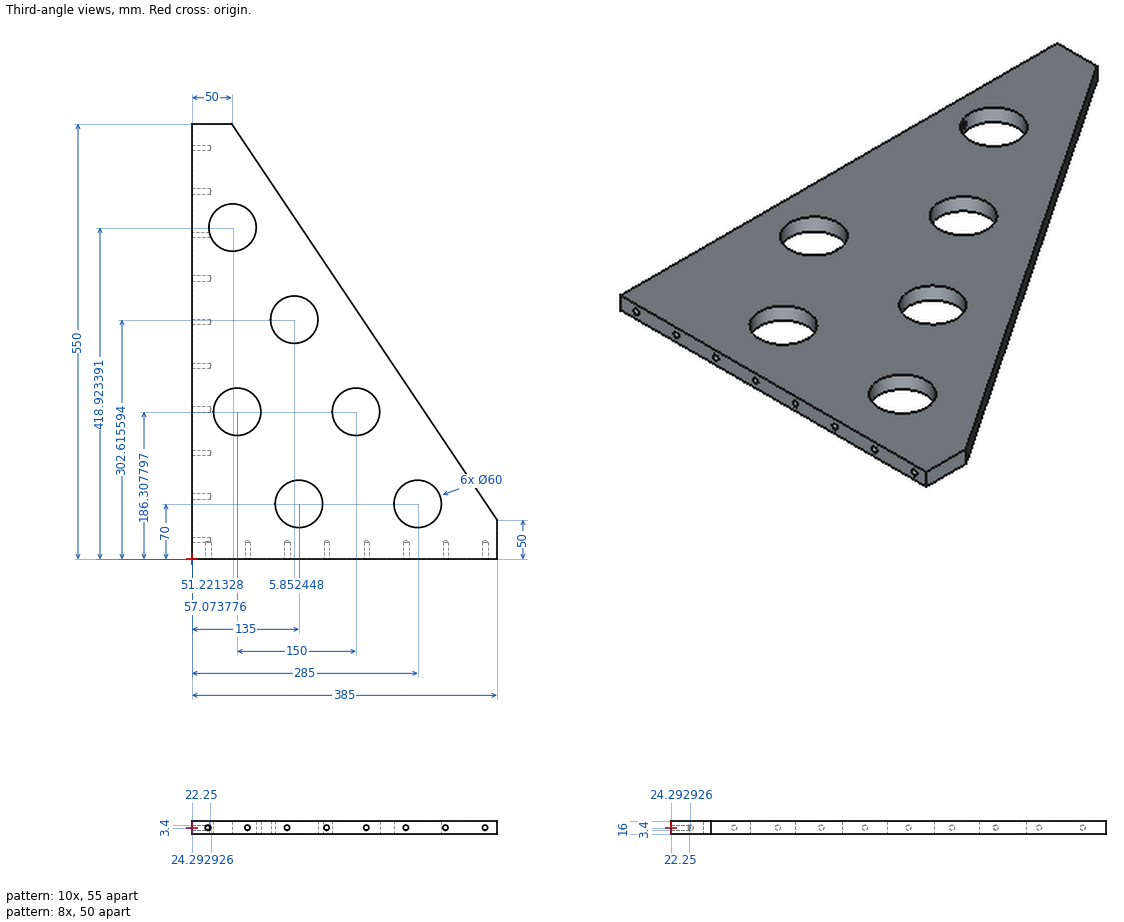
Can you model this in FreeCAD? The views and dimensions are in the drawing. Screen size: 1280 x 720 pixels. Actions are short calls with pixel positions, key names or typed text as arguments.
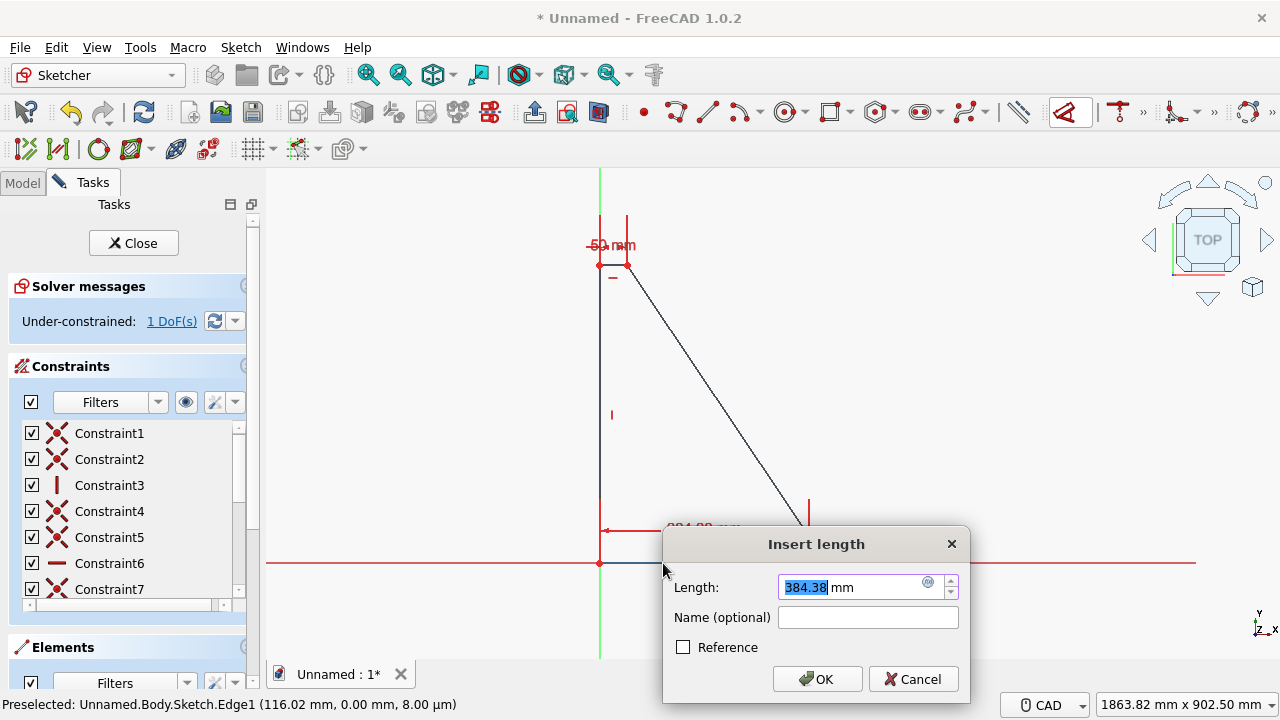
text(385)
key(Return)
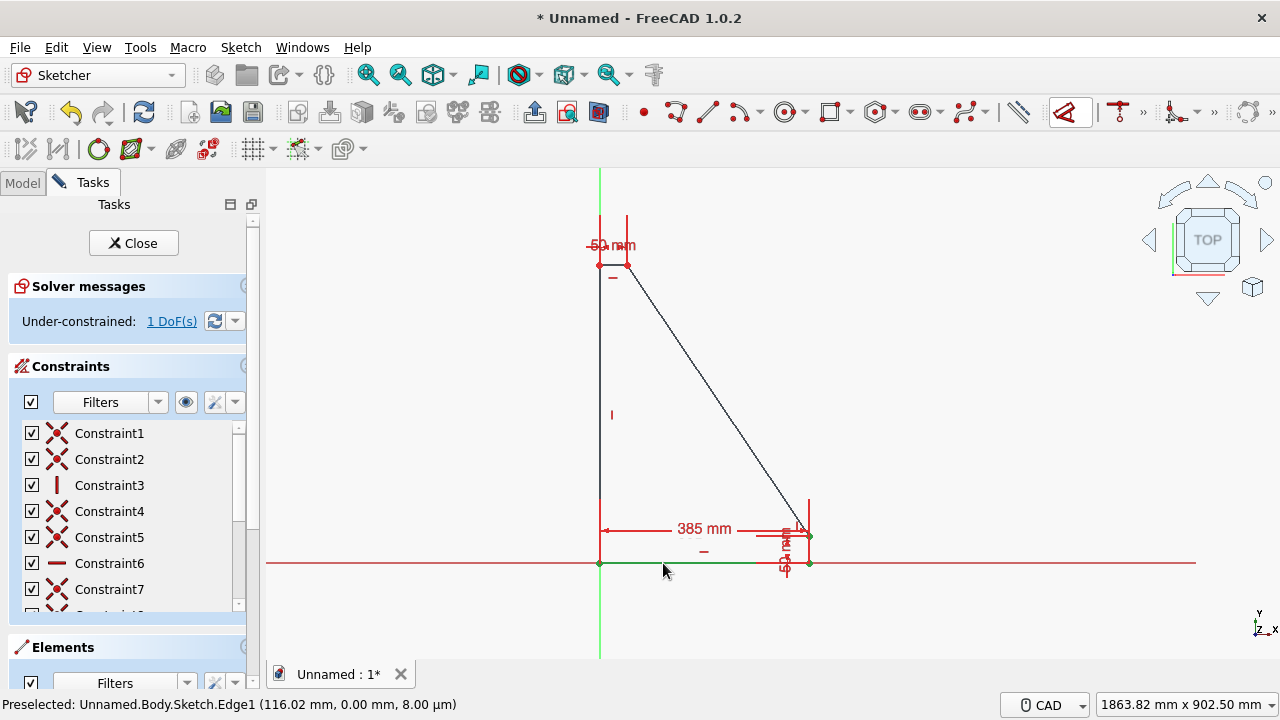
click(600, 355)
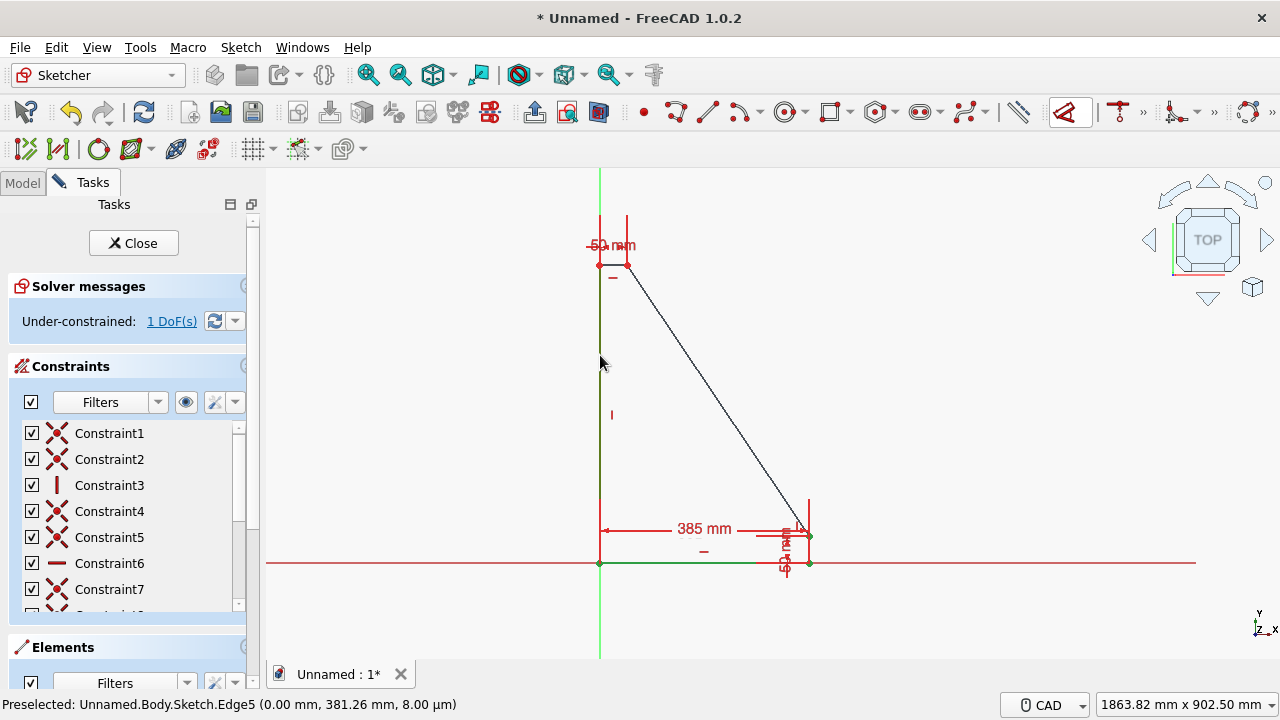
click(1086, 112)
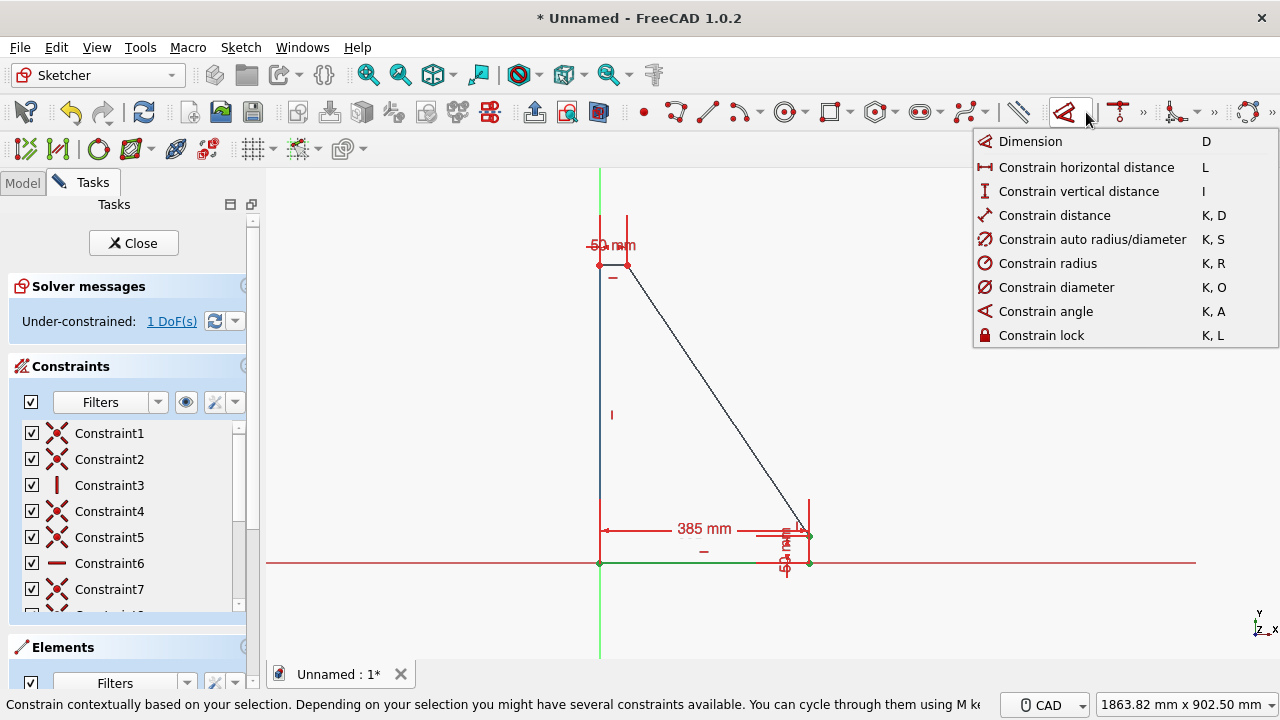
click(1126, 191)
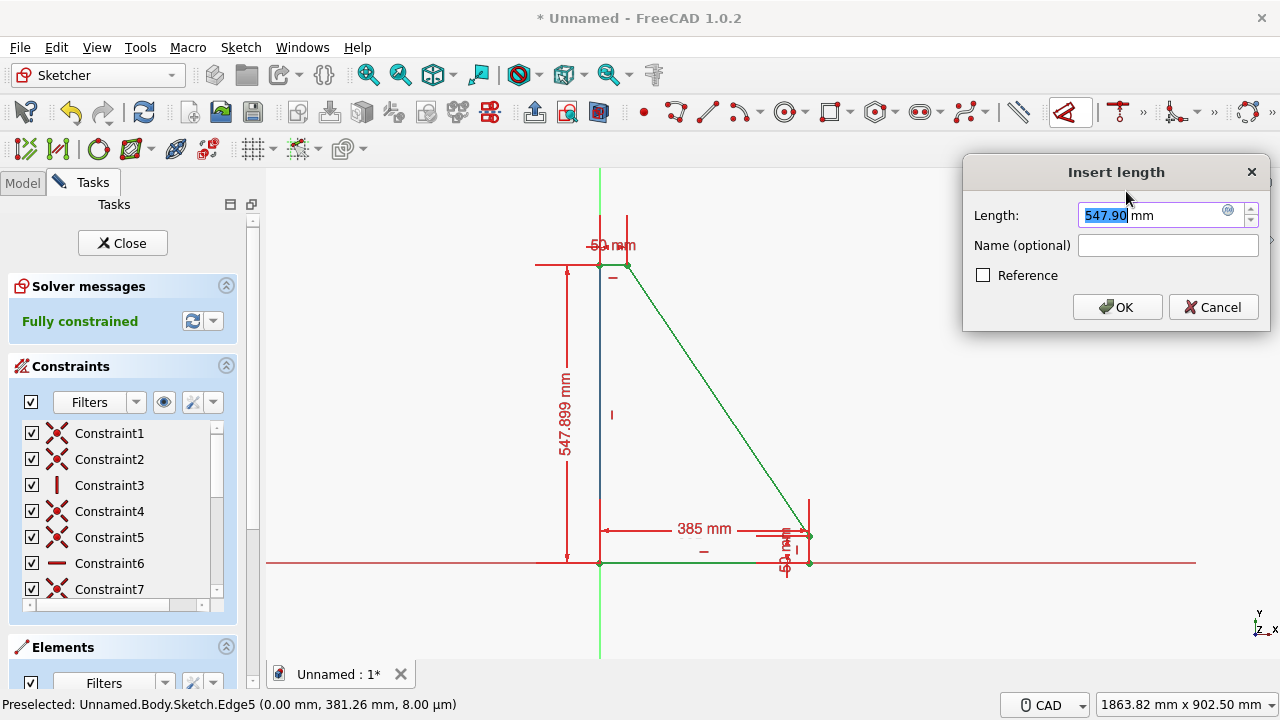
text(550)
key(Return)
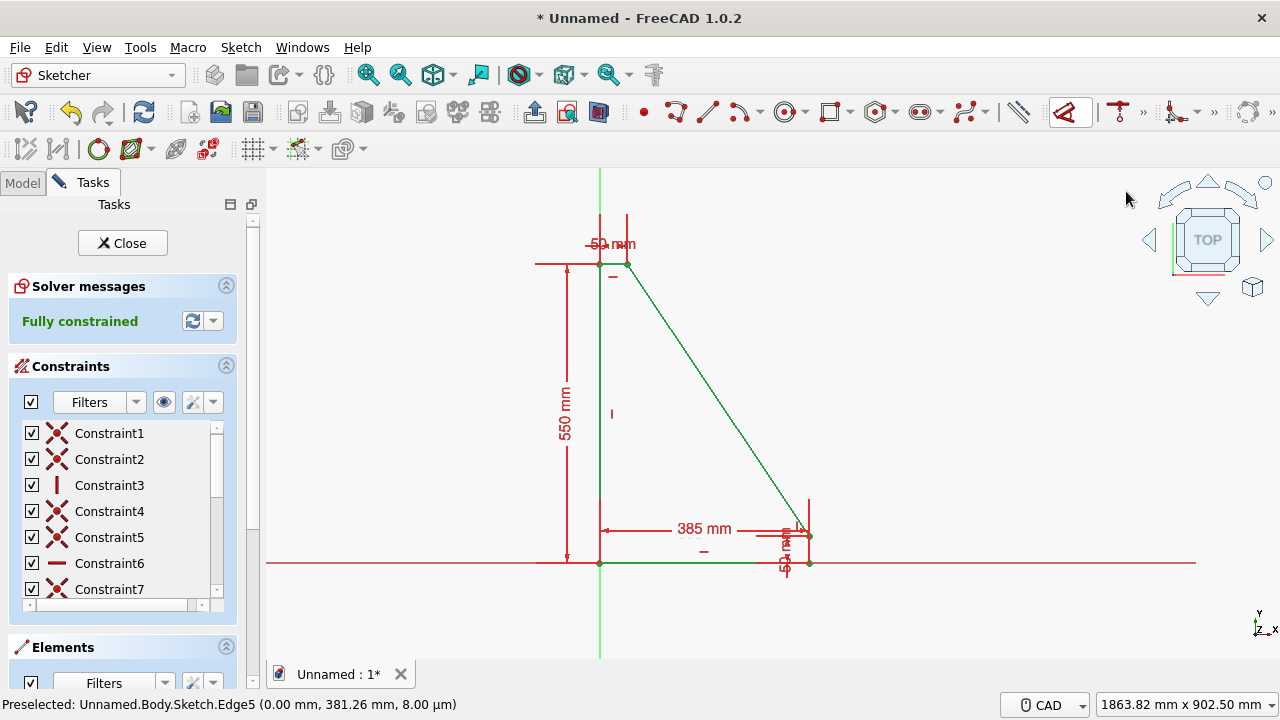
click(123, 243)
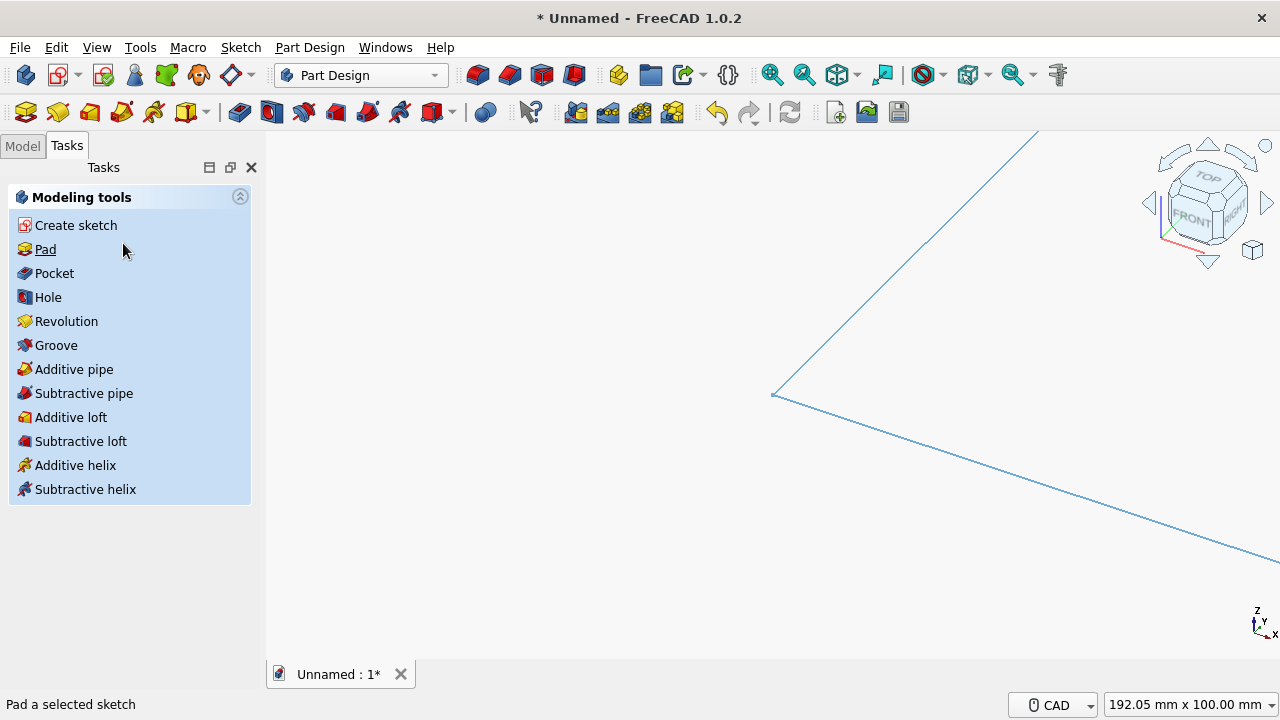
click(26, 112)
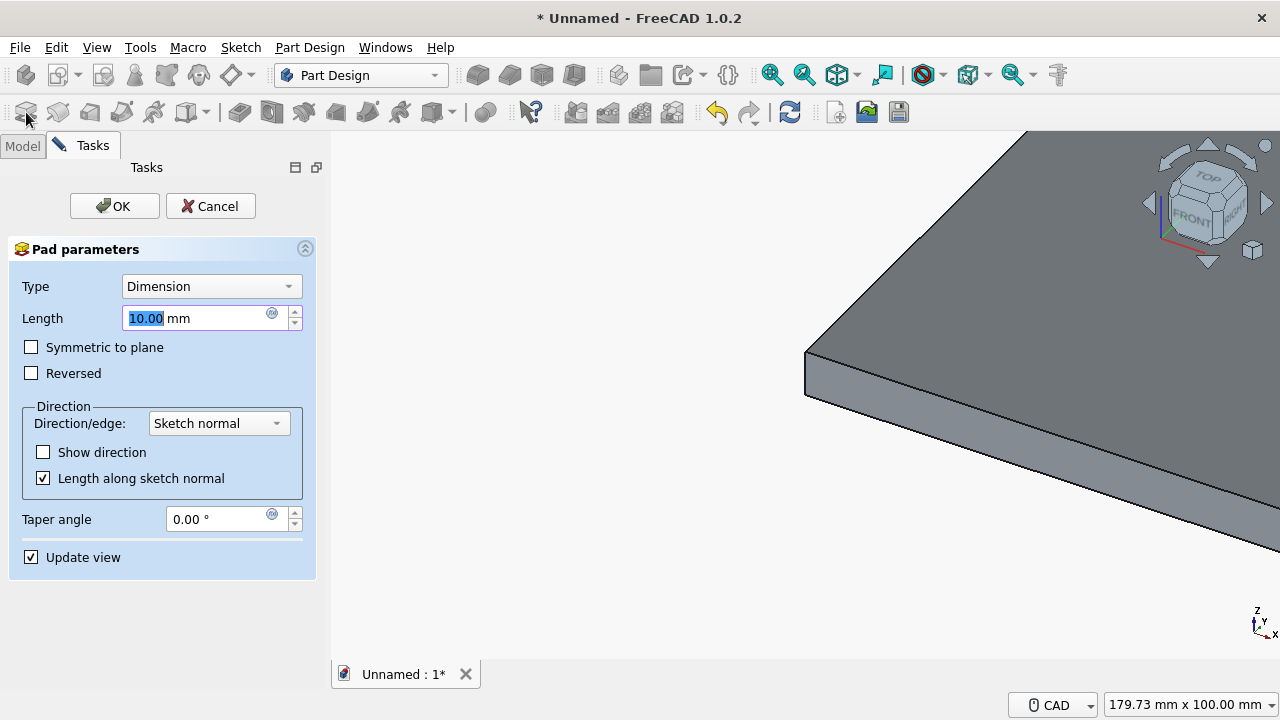
text(16)
key(Tab)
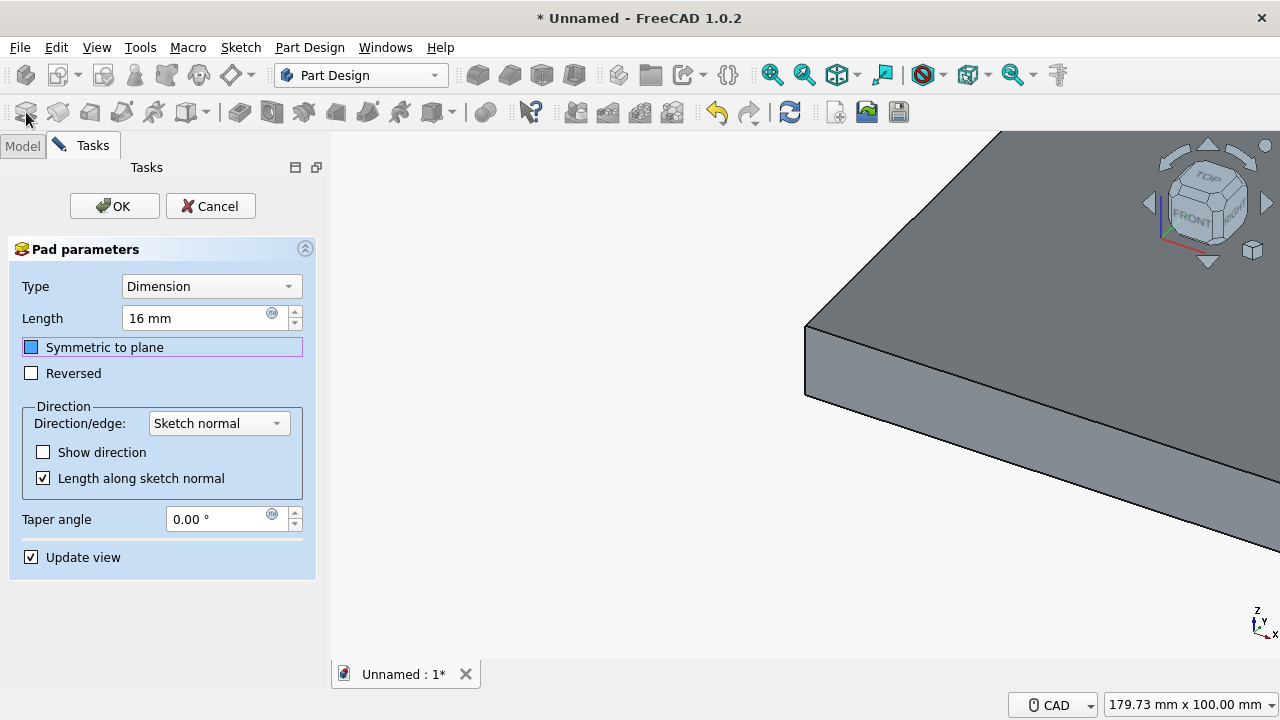
click(30, 347)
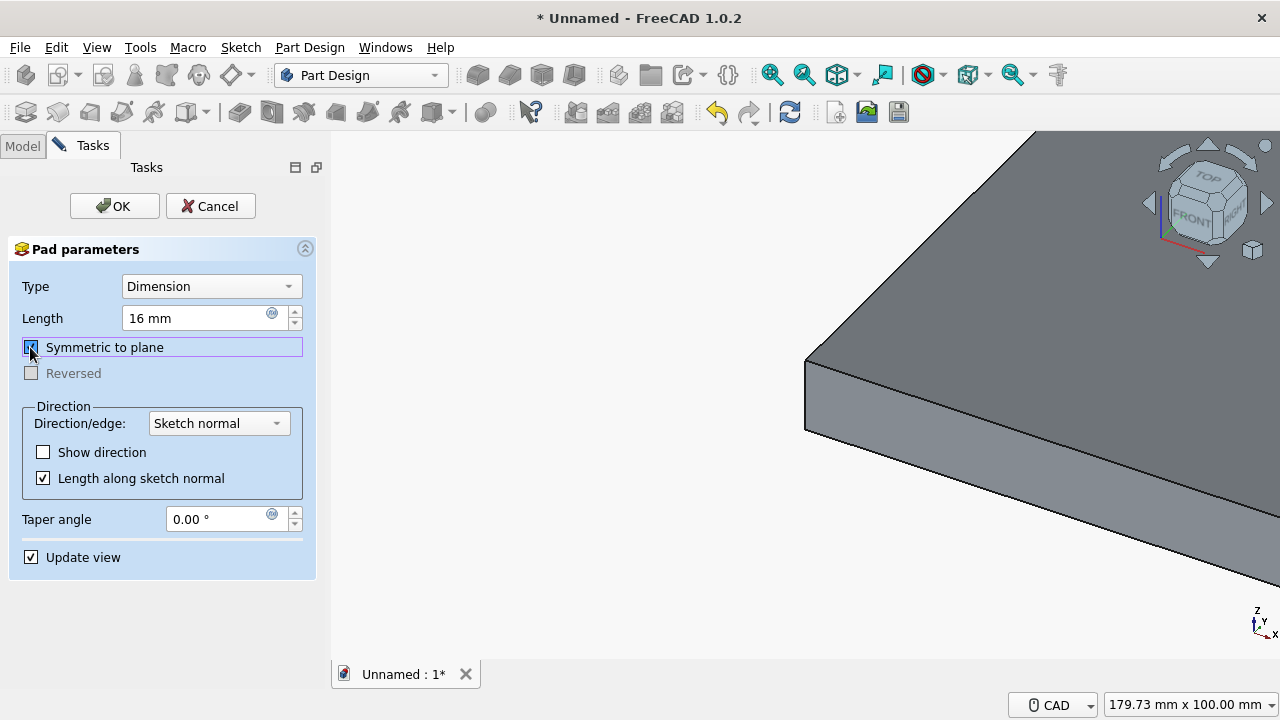
click(115, 206)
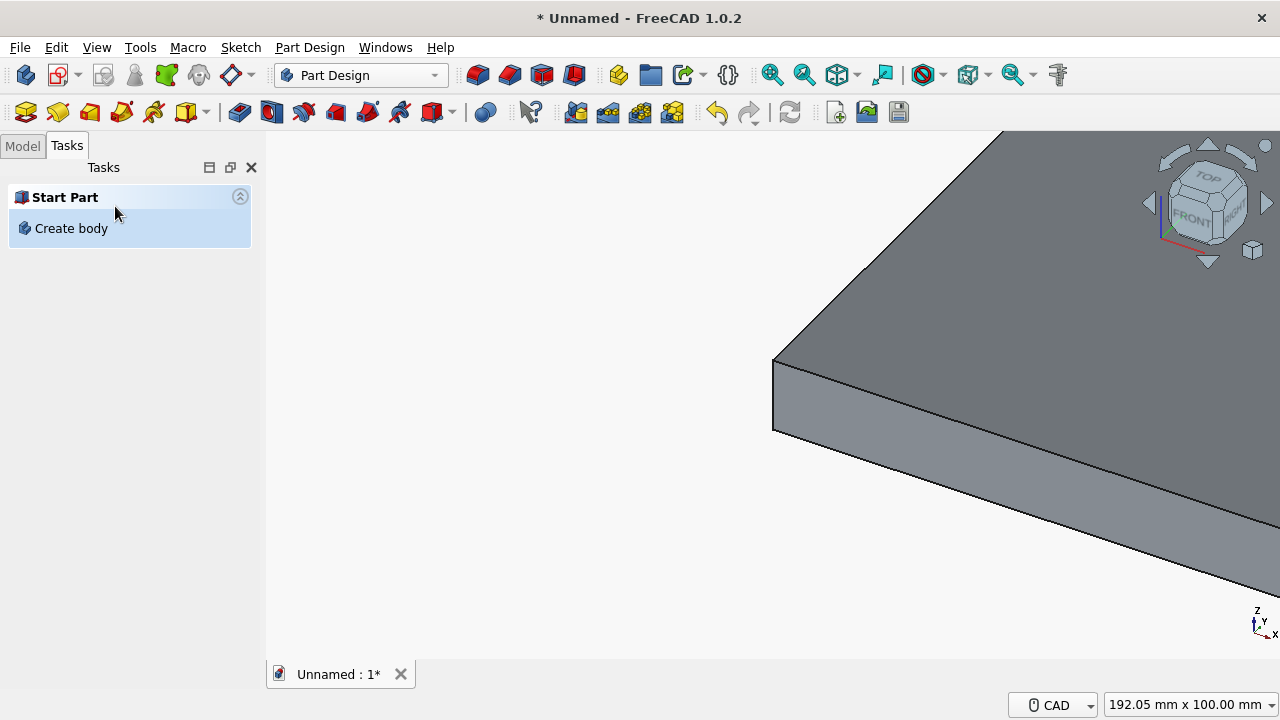
click(774, 76)